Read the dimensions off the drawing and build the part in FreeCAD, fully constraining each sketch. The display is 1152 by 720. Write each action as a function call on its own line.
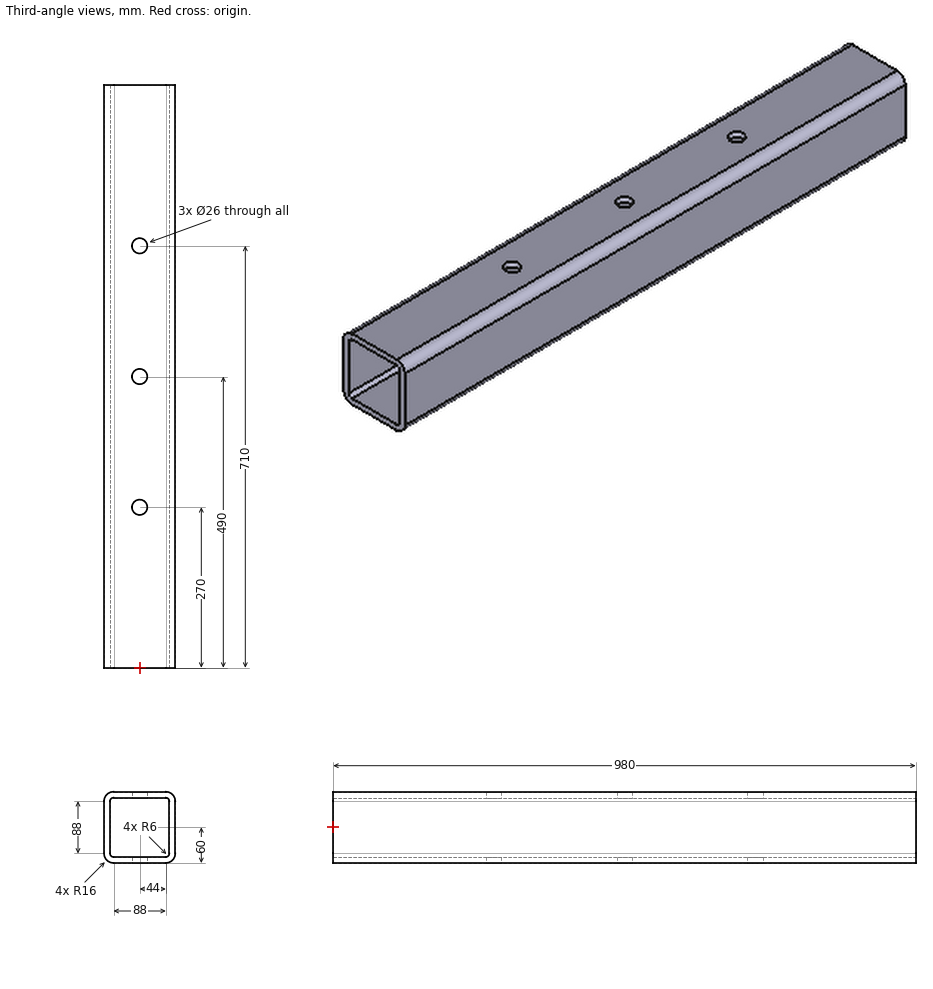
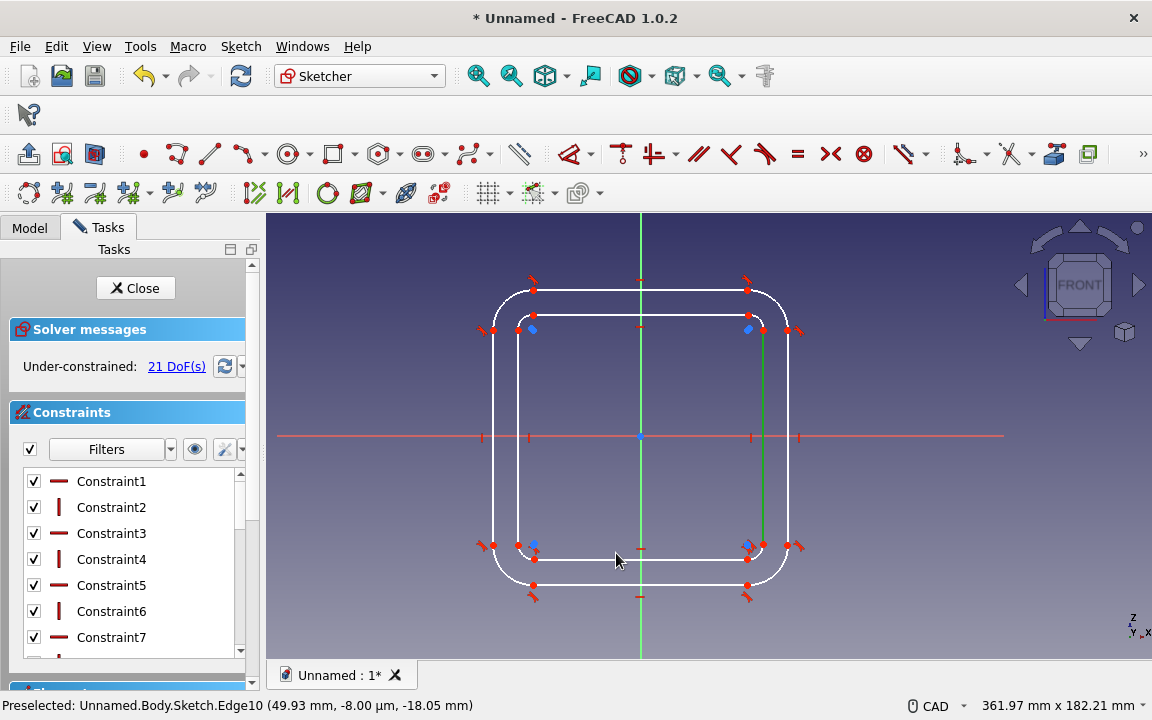
scroll(762, 323, up, 4)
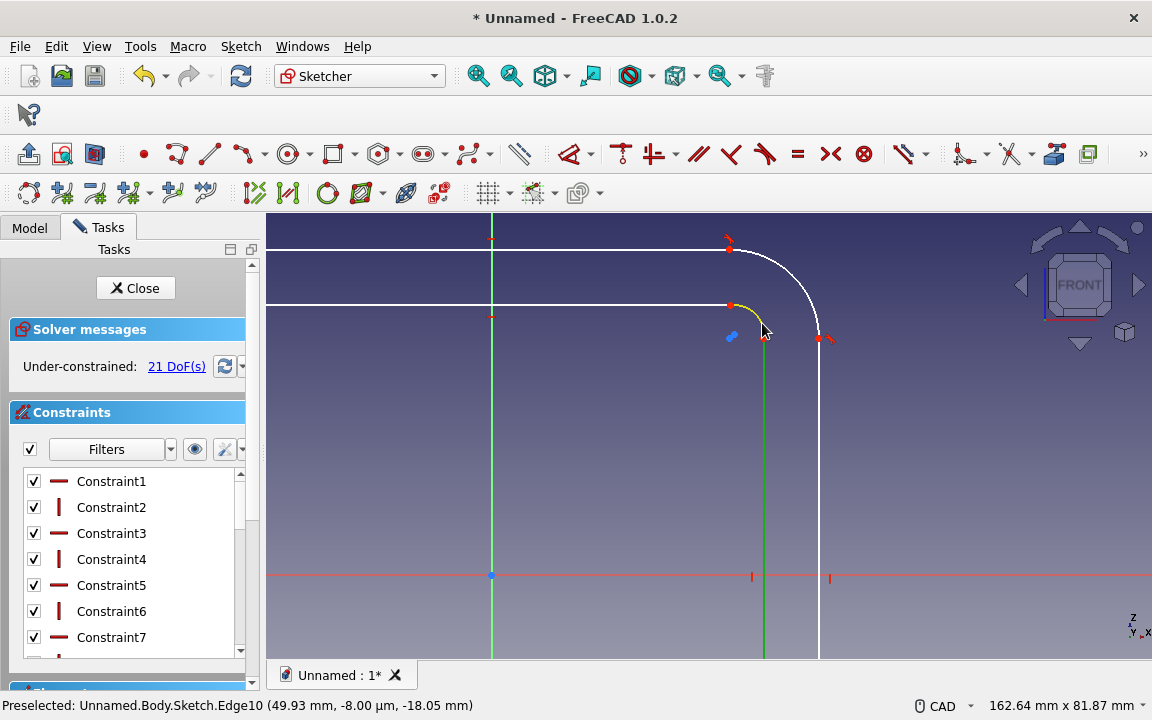
click(761, 323)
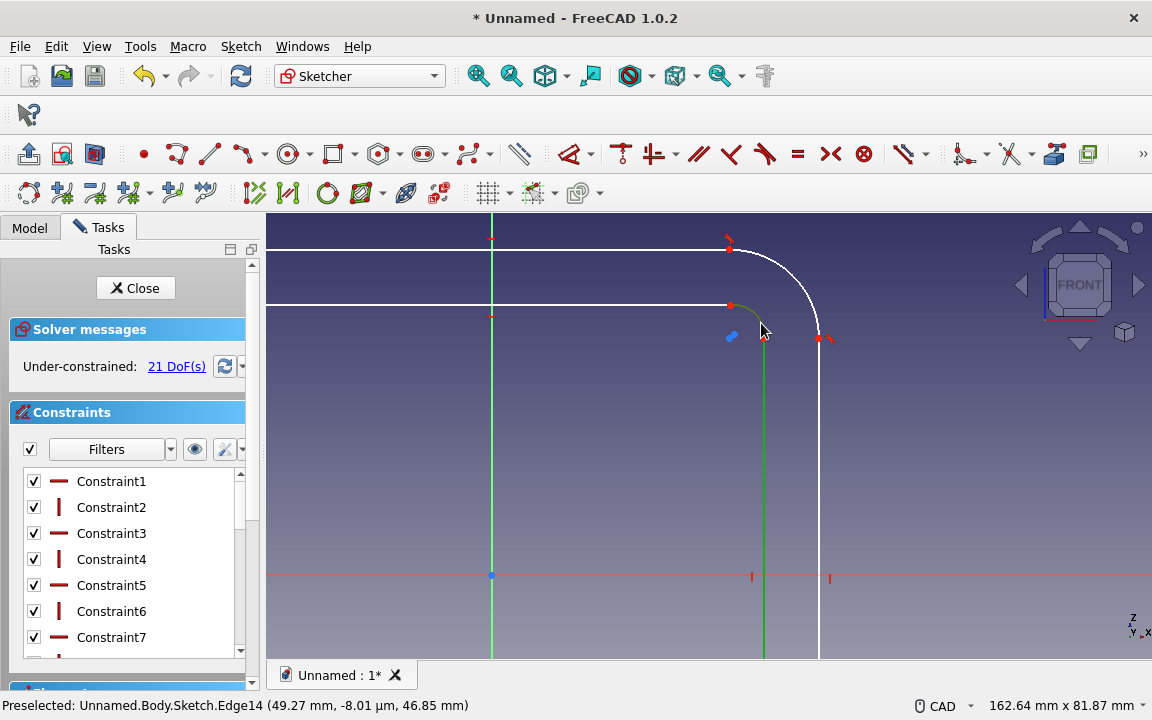
click(765, 154)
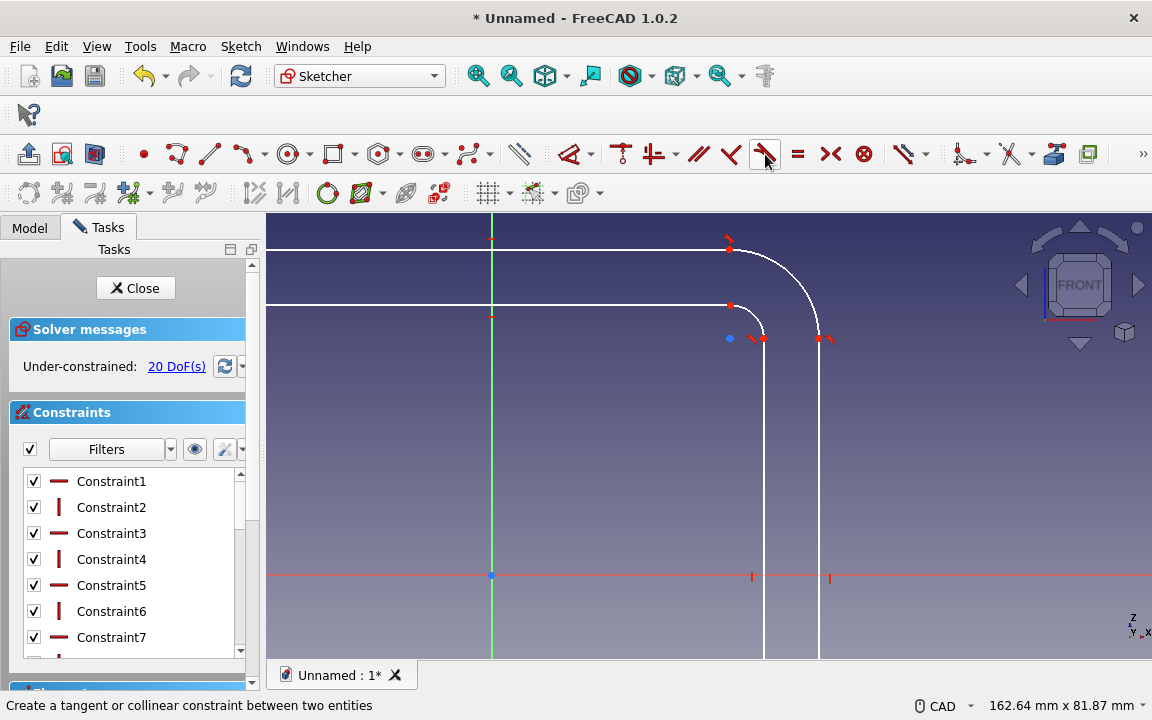
click(587, 305)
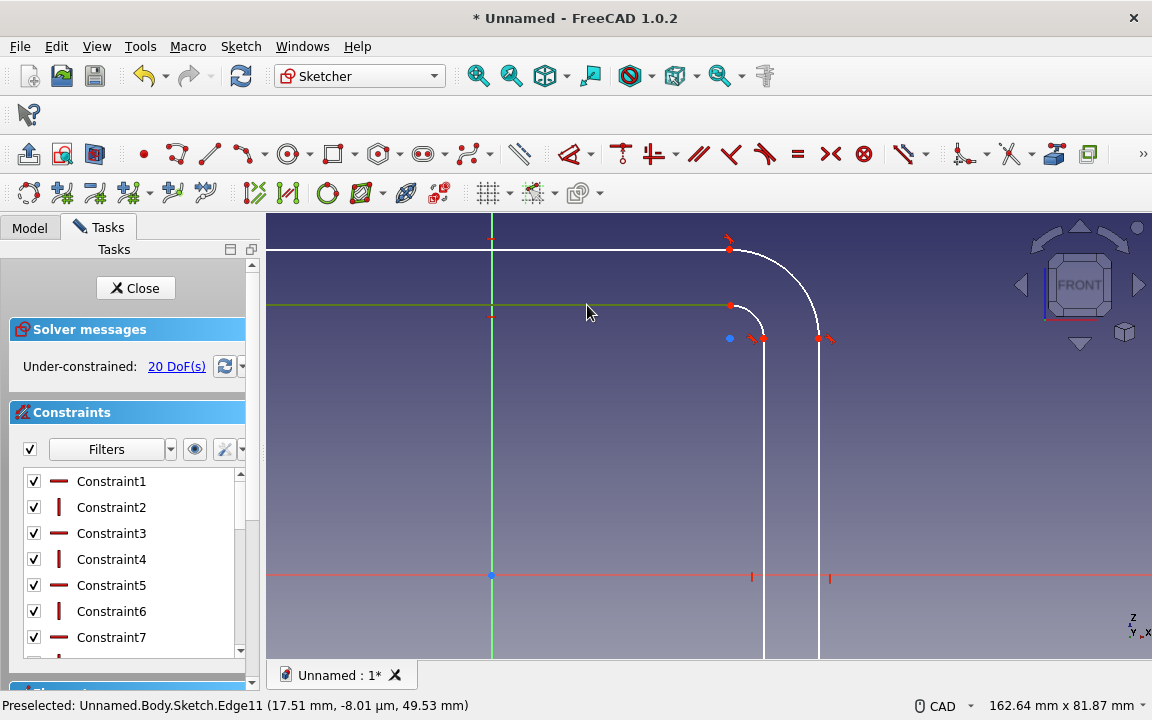
click(760, 324)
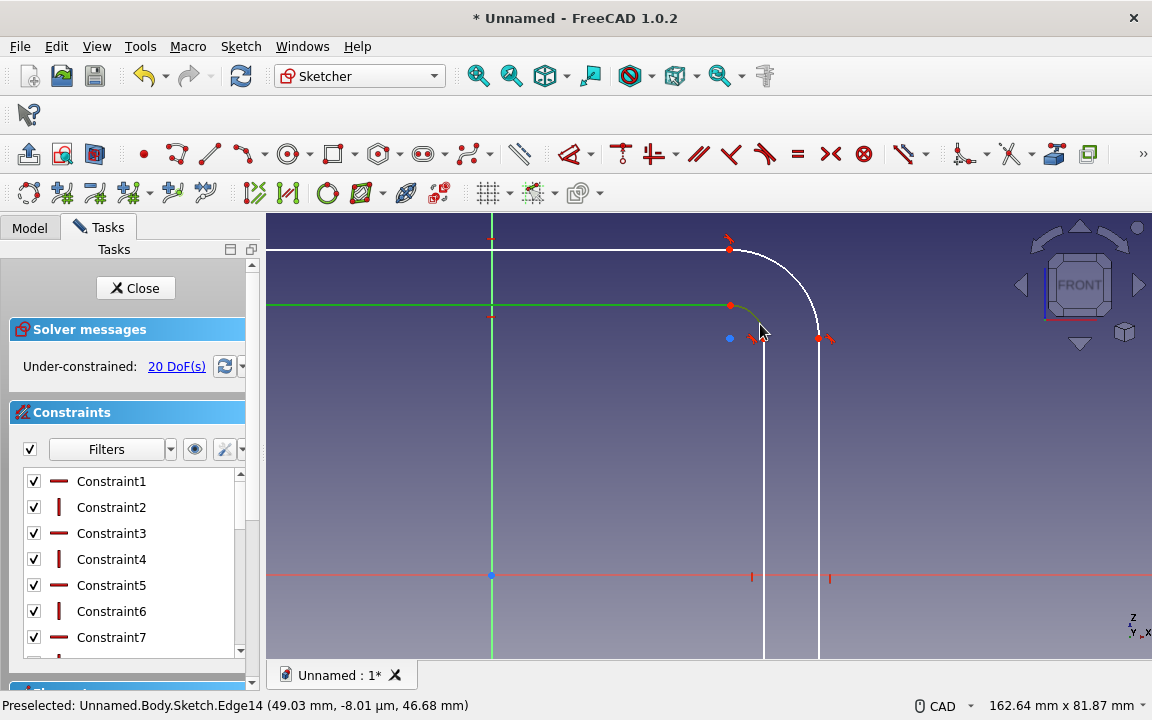
click(765, 154)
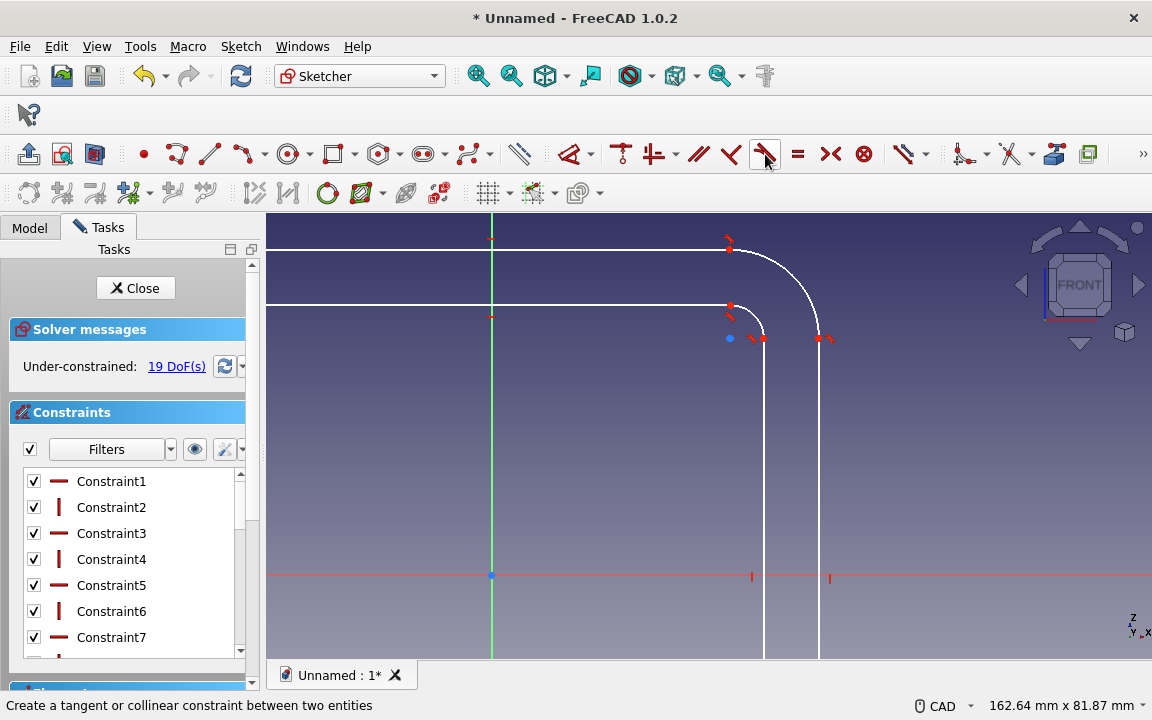
click(587, 305)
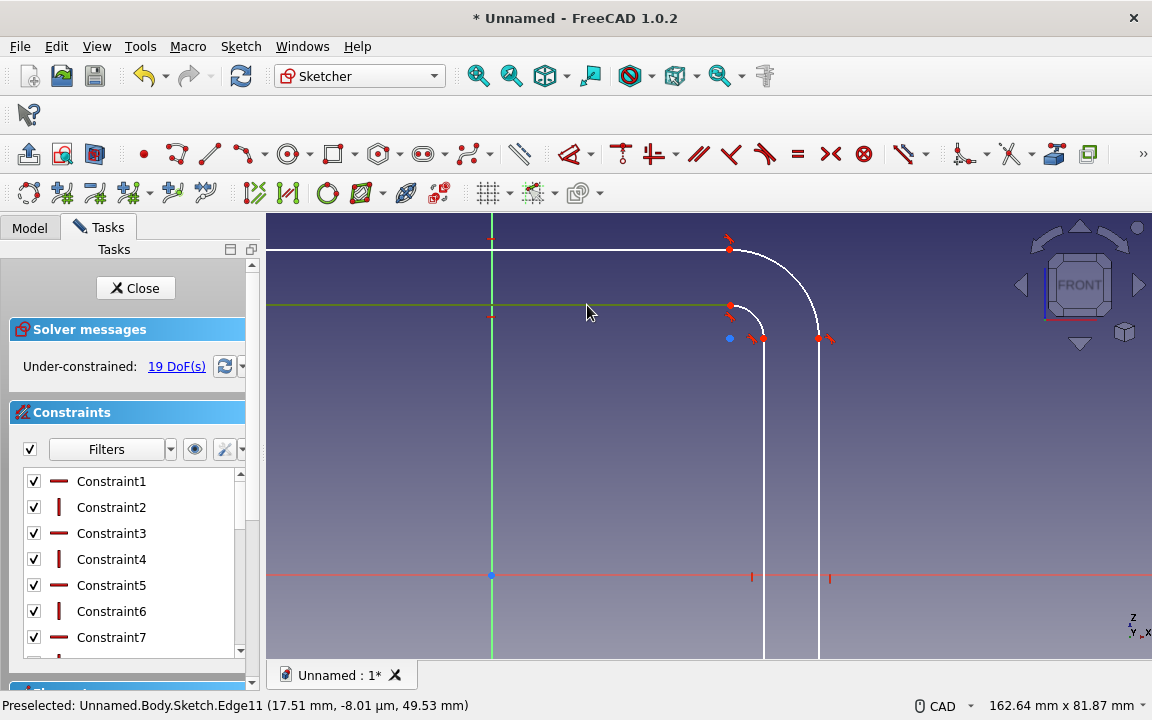
scroll(762, 322, down, 4)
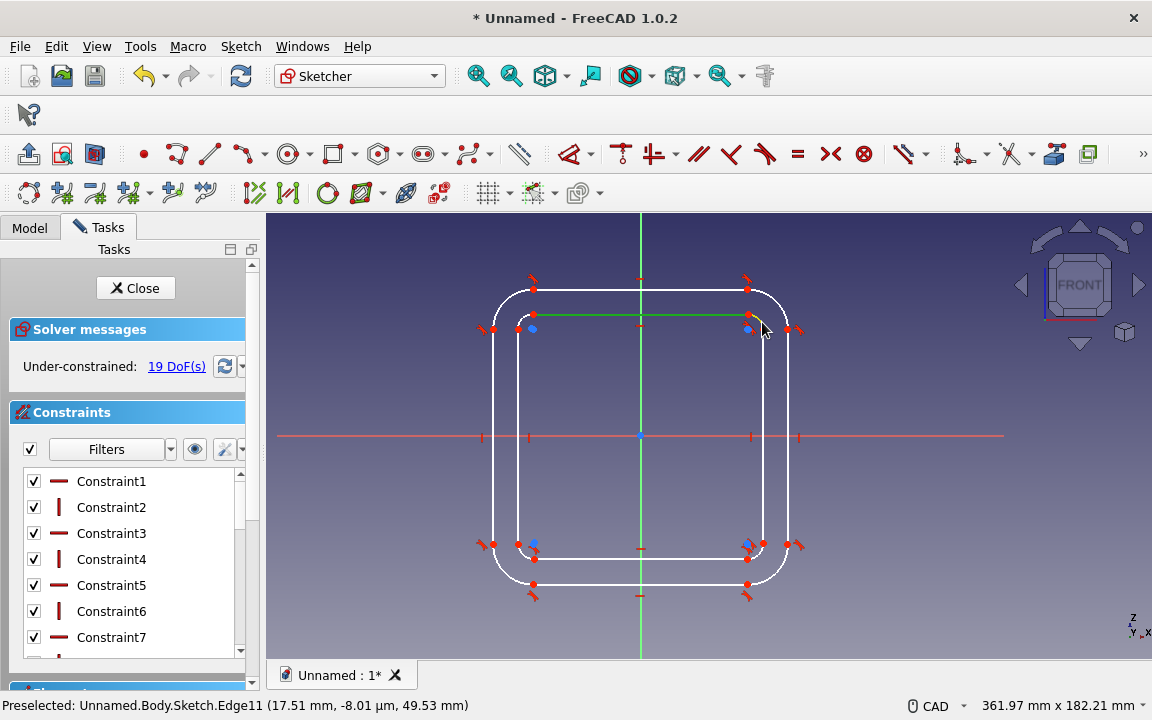
scroll(526, 316, up, 4)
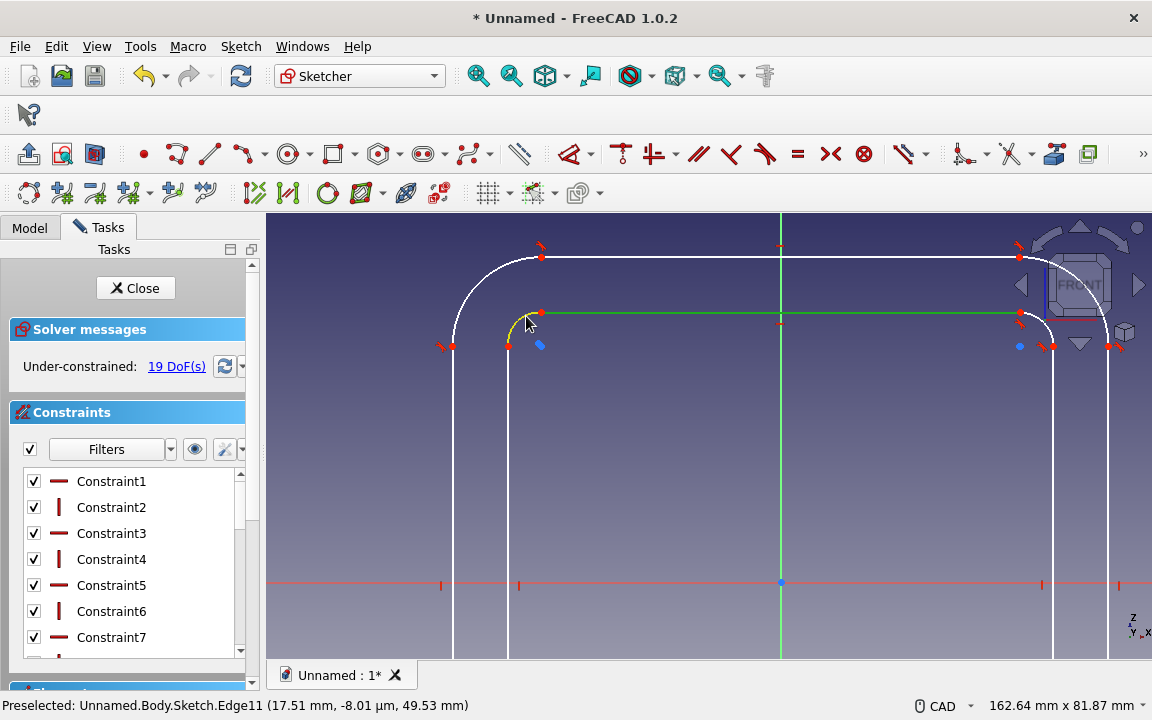
click(526, 315)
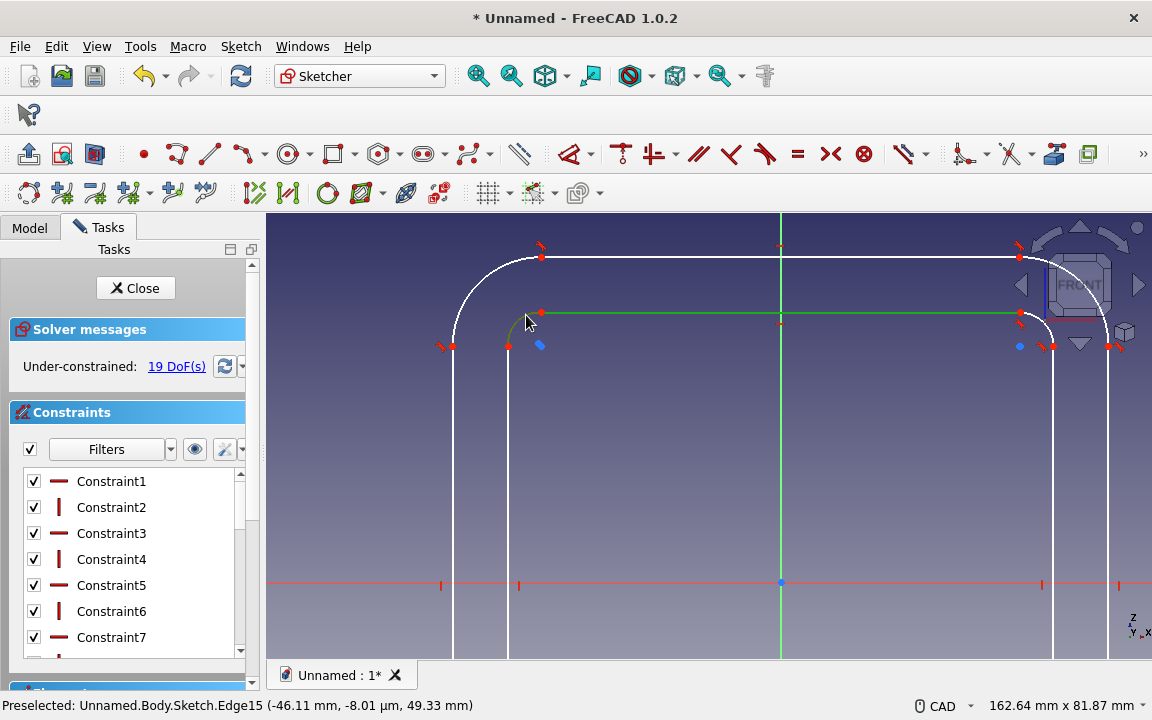
click(765, 154)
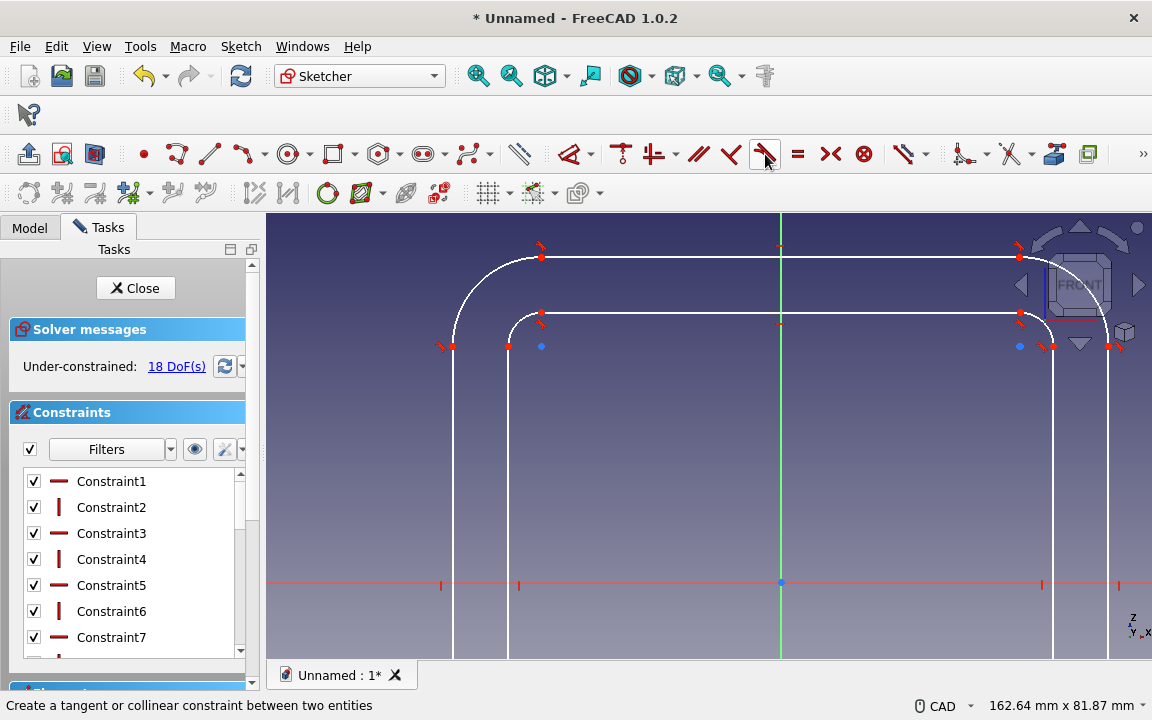
click(508, 490)